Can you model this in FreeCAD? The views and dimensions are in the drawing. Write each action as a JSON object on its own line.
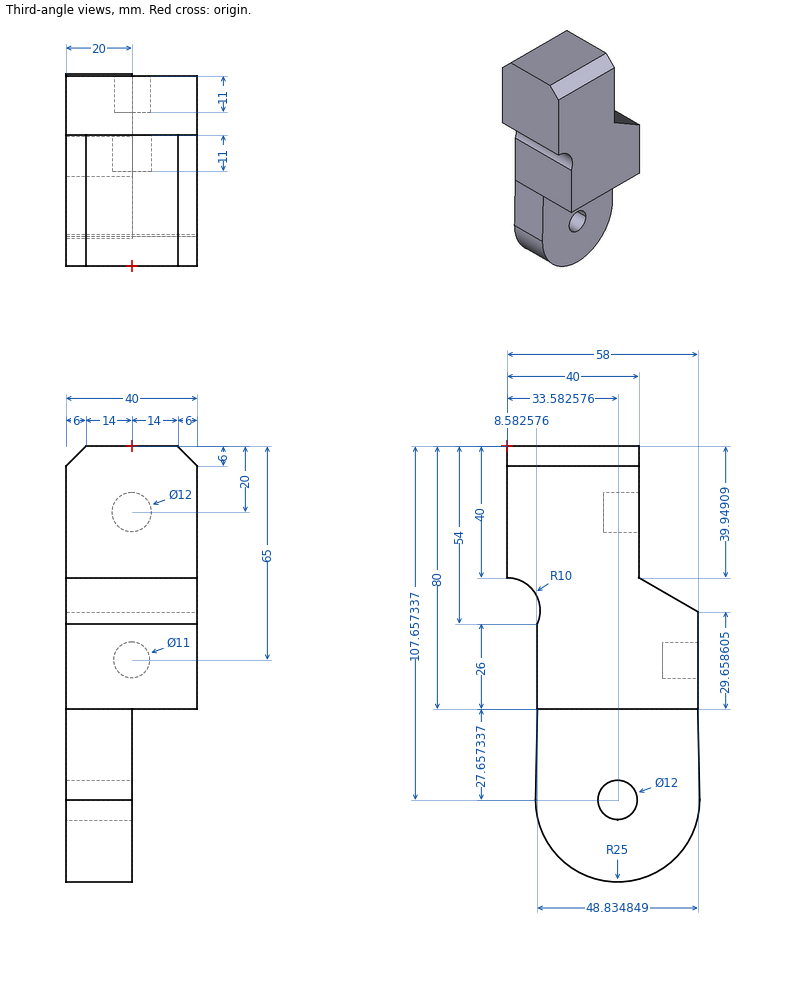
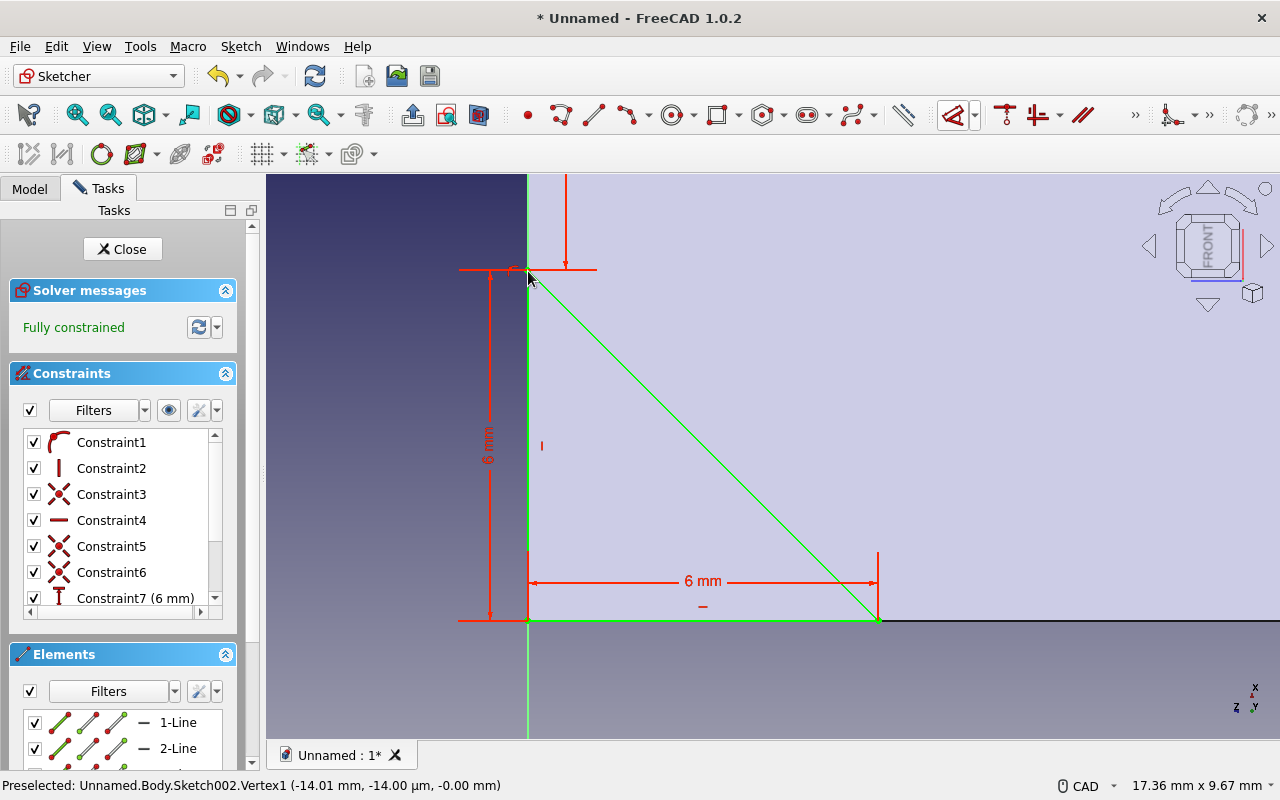
{"action": "left_click", "coordinate": [123, 249]}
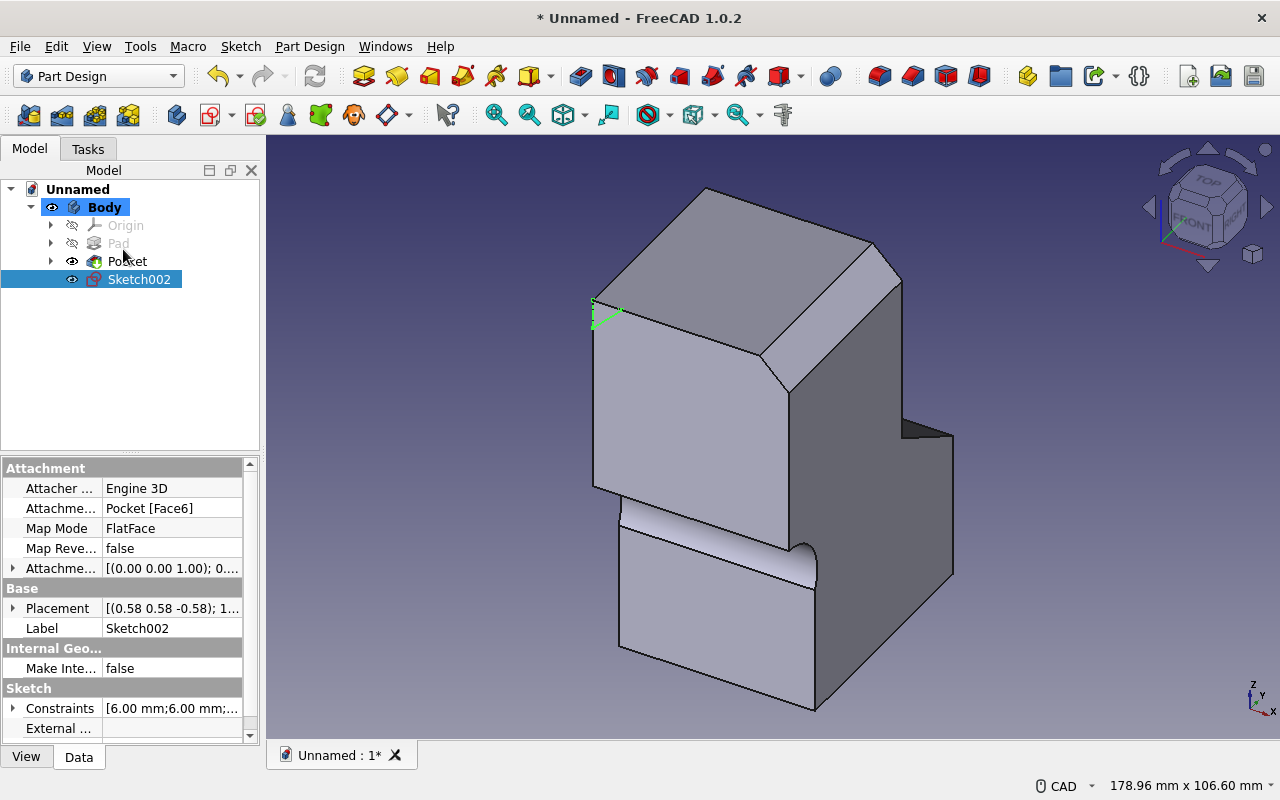
{"action": "left_click", "coordinate": [581, 76]}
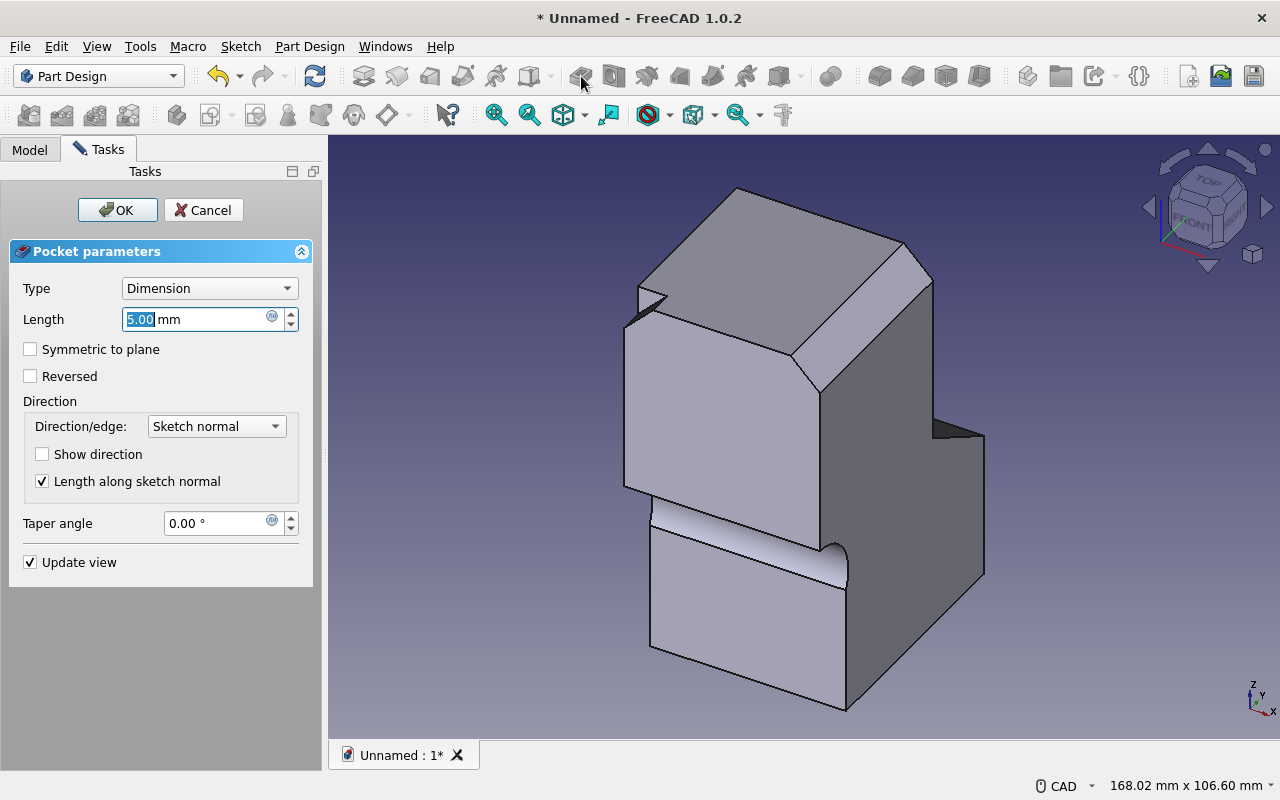
{"action": "left_click", "coordinate": [210, 288]}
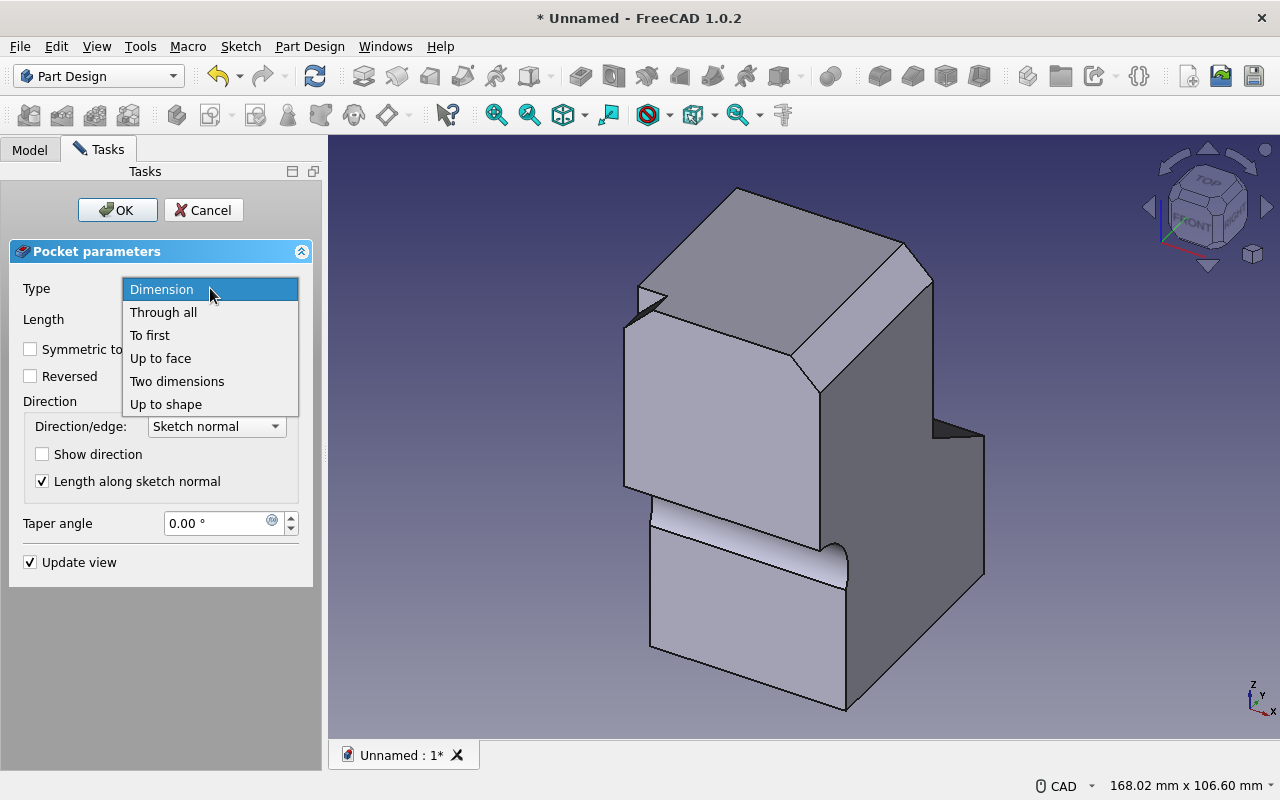
{"action": "left_click", "coordinate": [208, 312]}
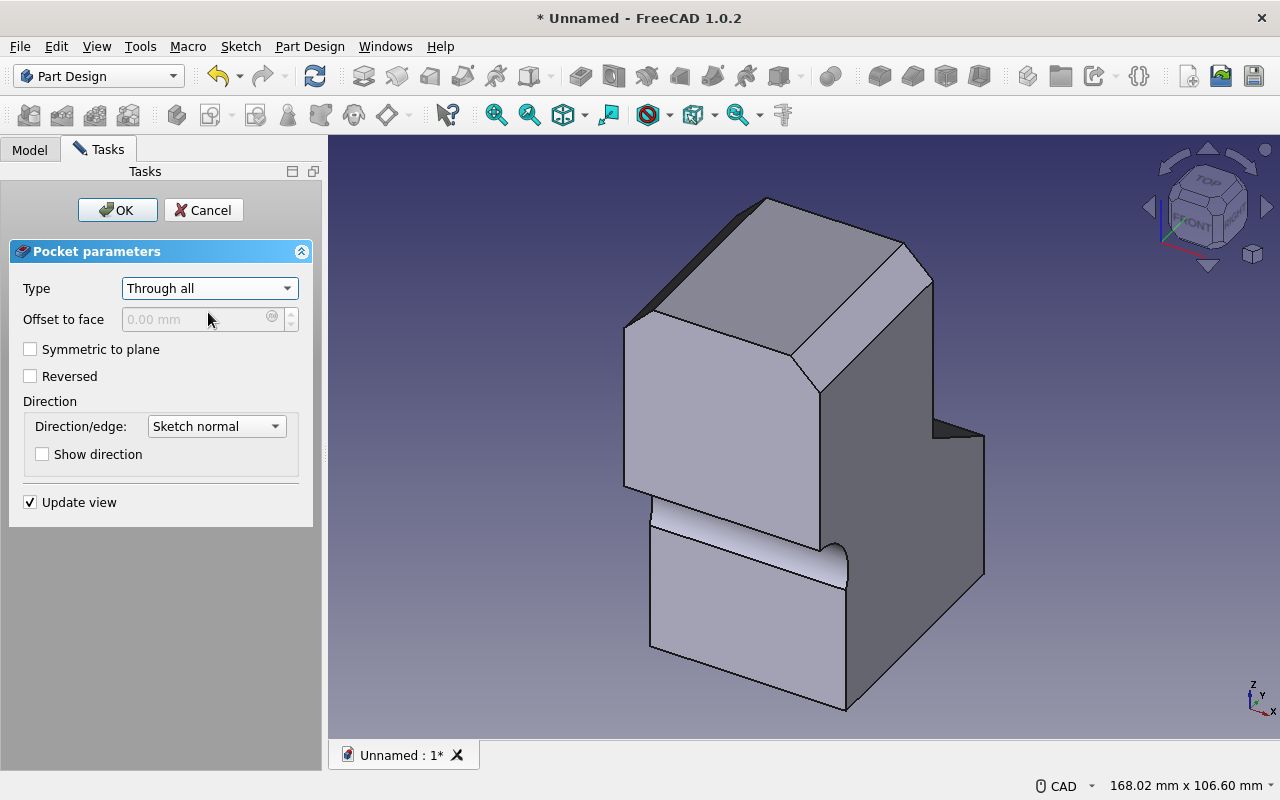
{"action": "left_click", "coordinate": [118, 210]}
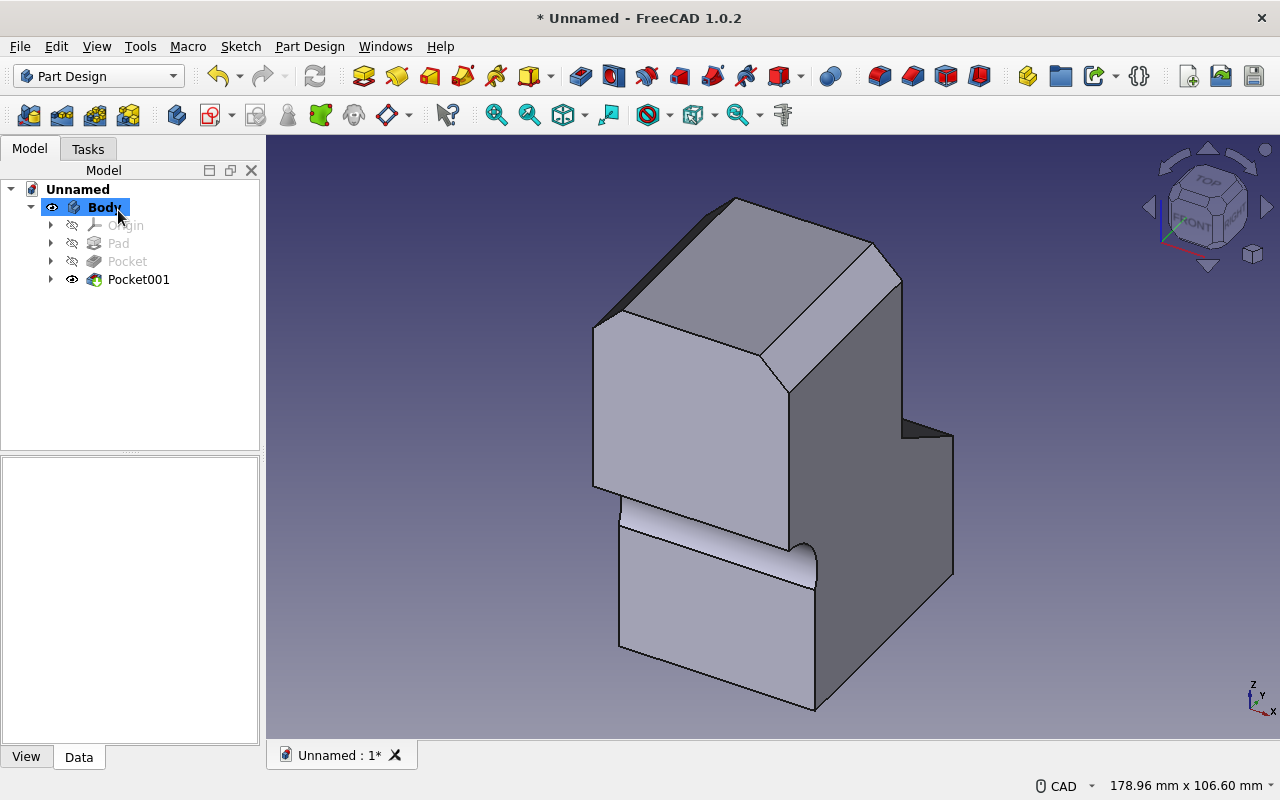
{"action": "key", "text": "4"}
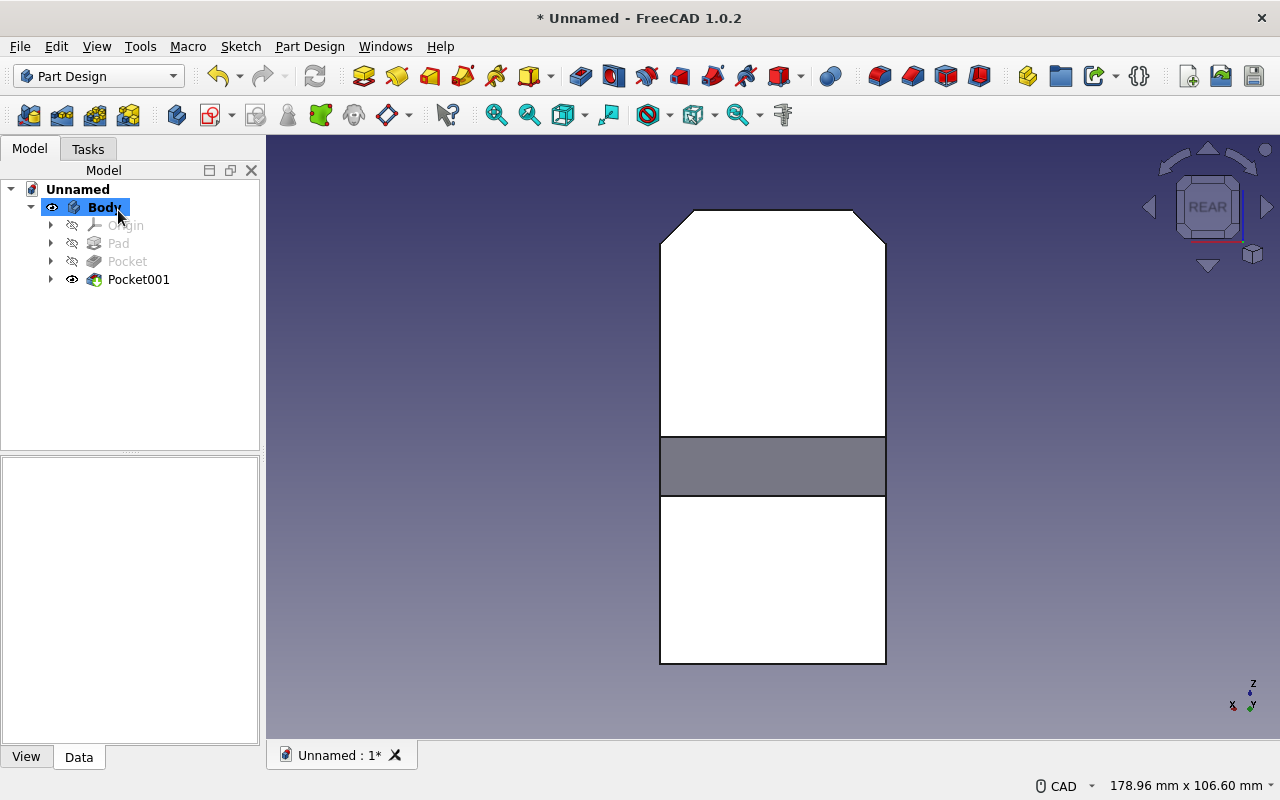
{"action": "left_click", "coordinate": [773, 323]}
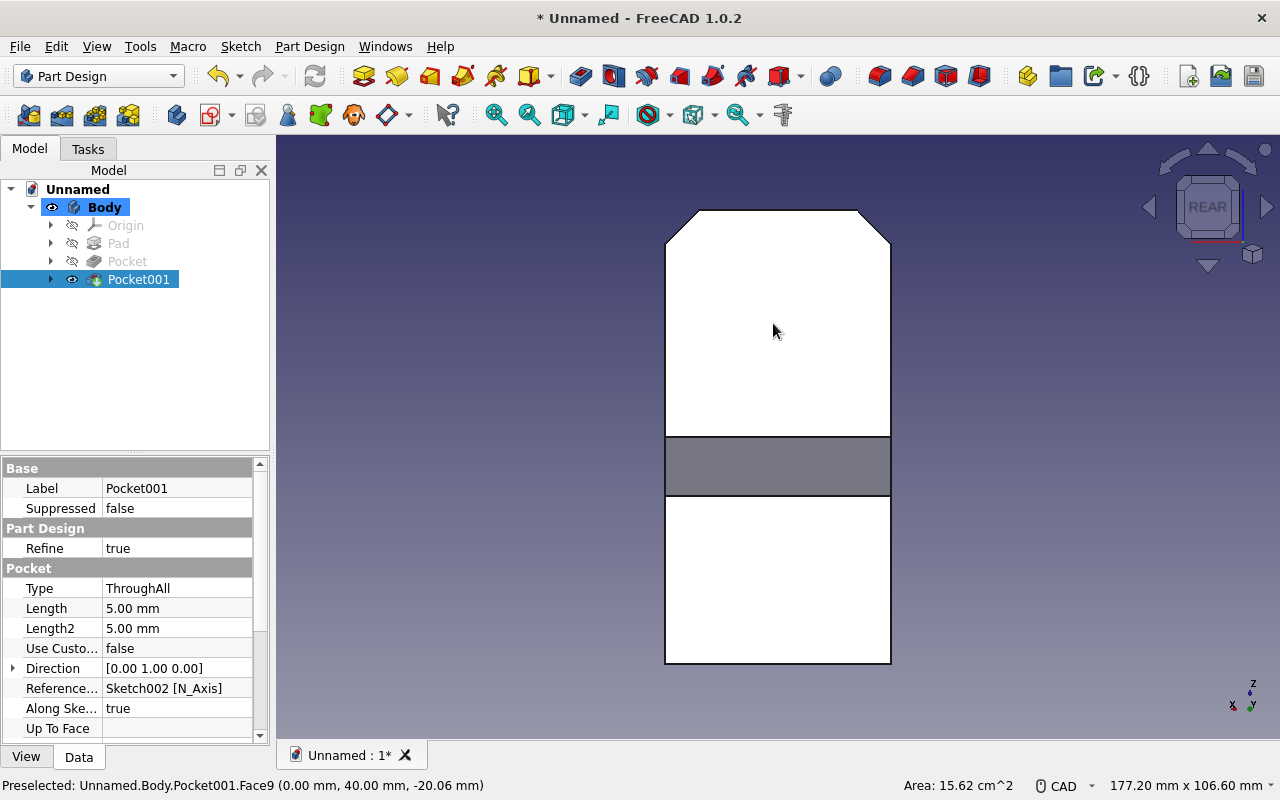
{"action": "left_click", "coordinate": [210, 116]}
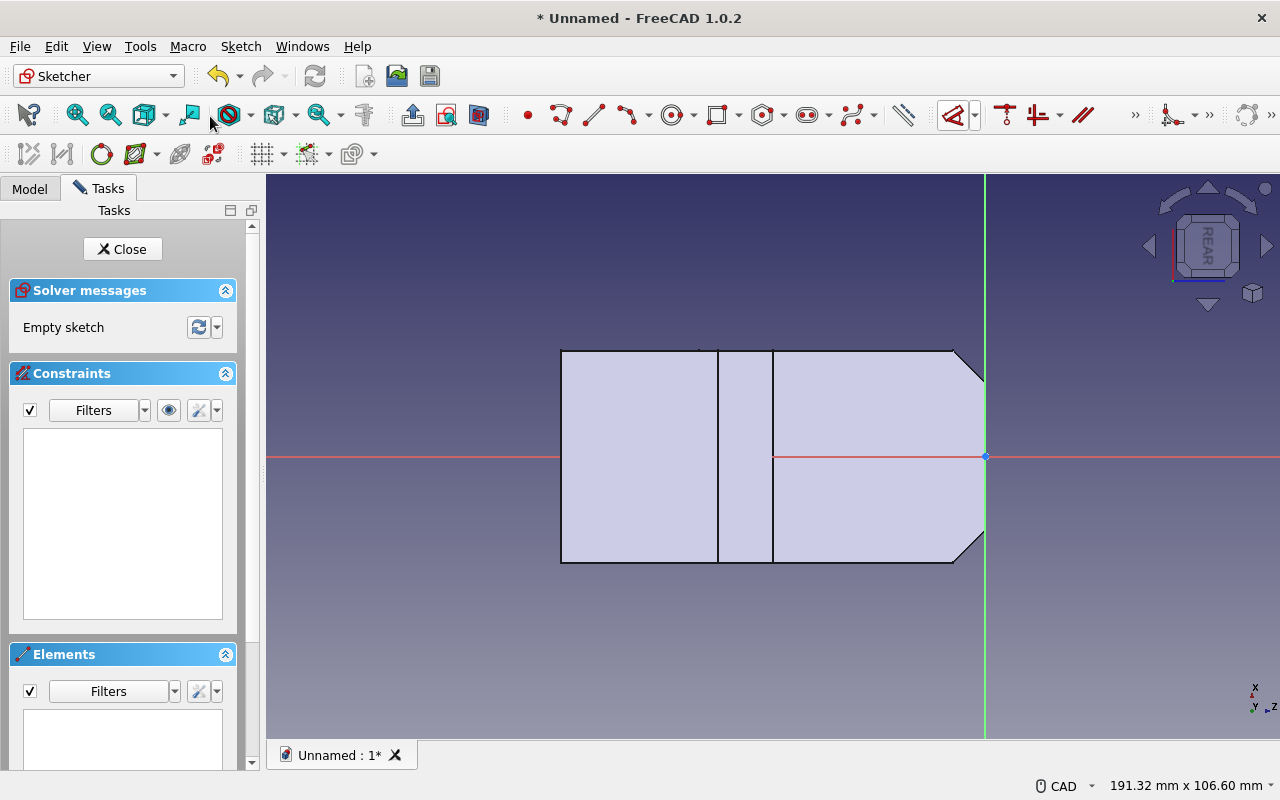
{"action": "left_click", "coordinate": [479, 116]}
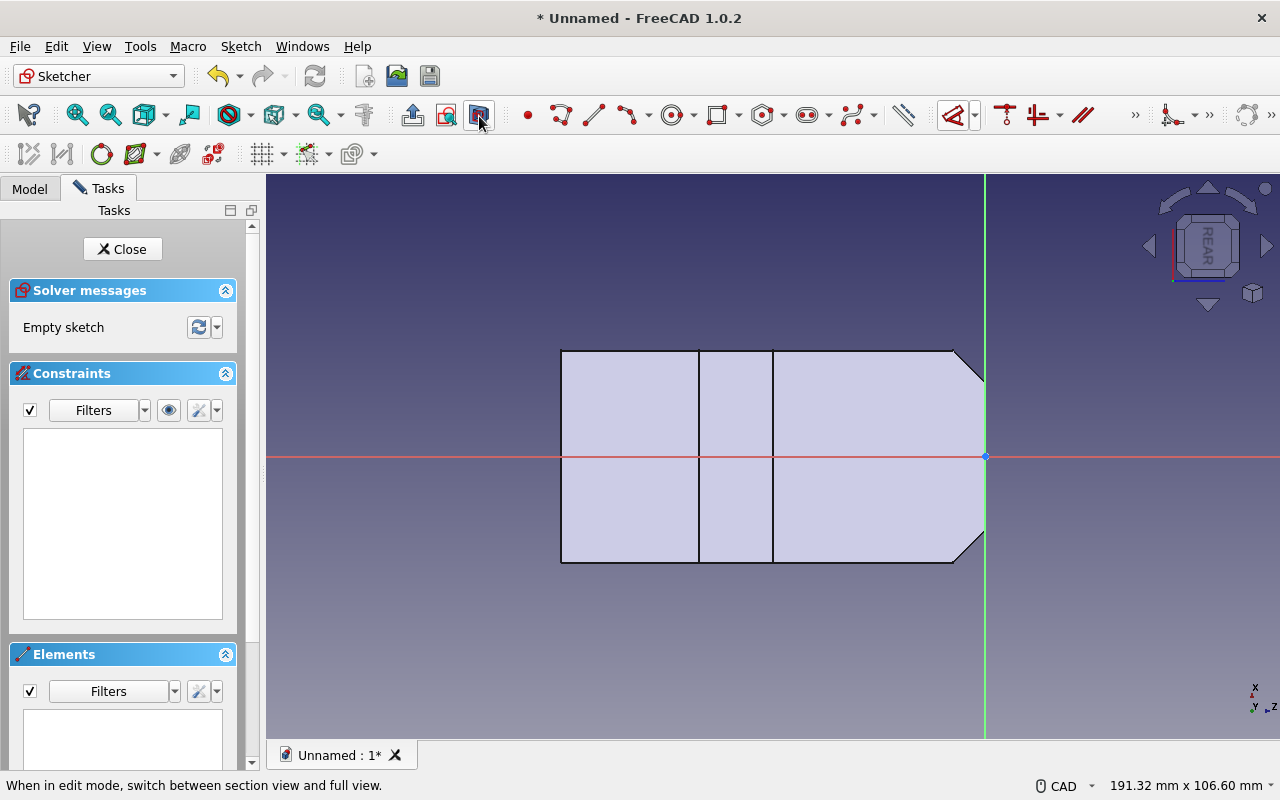
{"action": "scroll", "coordinate": [985, 456], "scroll_direction": "up", "scroll_amount": 7}